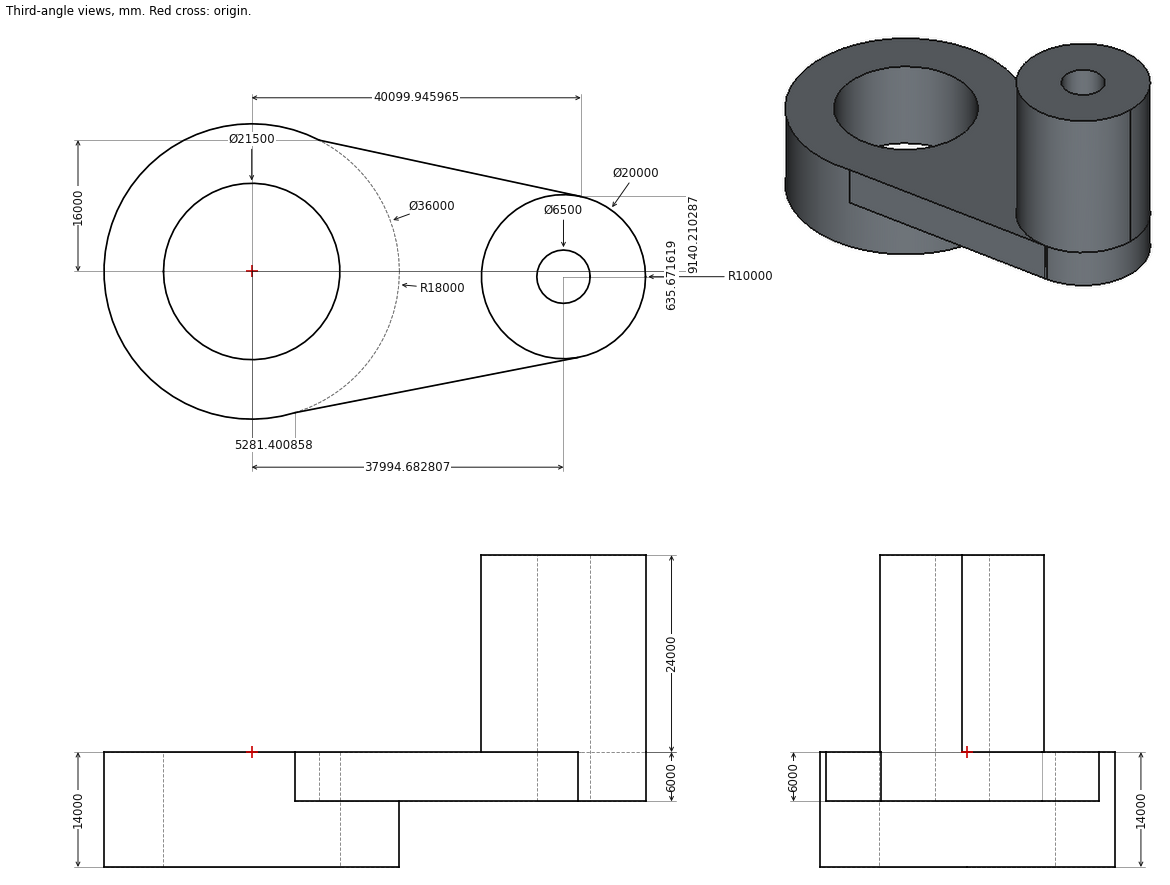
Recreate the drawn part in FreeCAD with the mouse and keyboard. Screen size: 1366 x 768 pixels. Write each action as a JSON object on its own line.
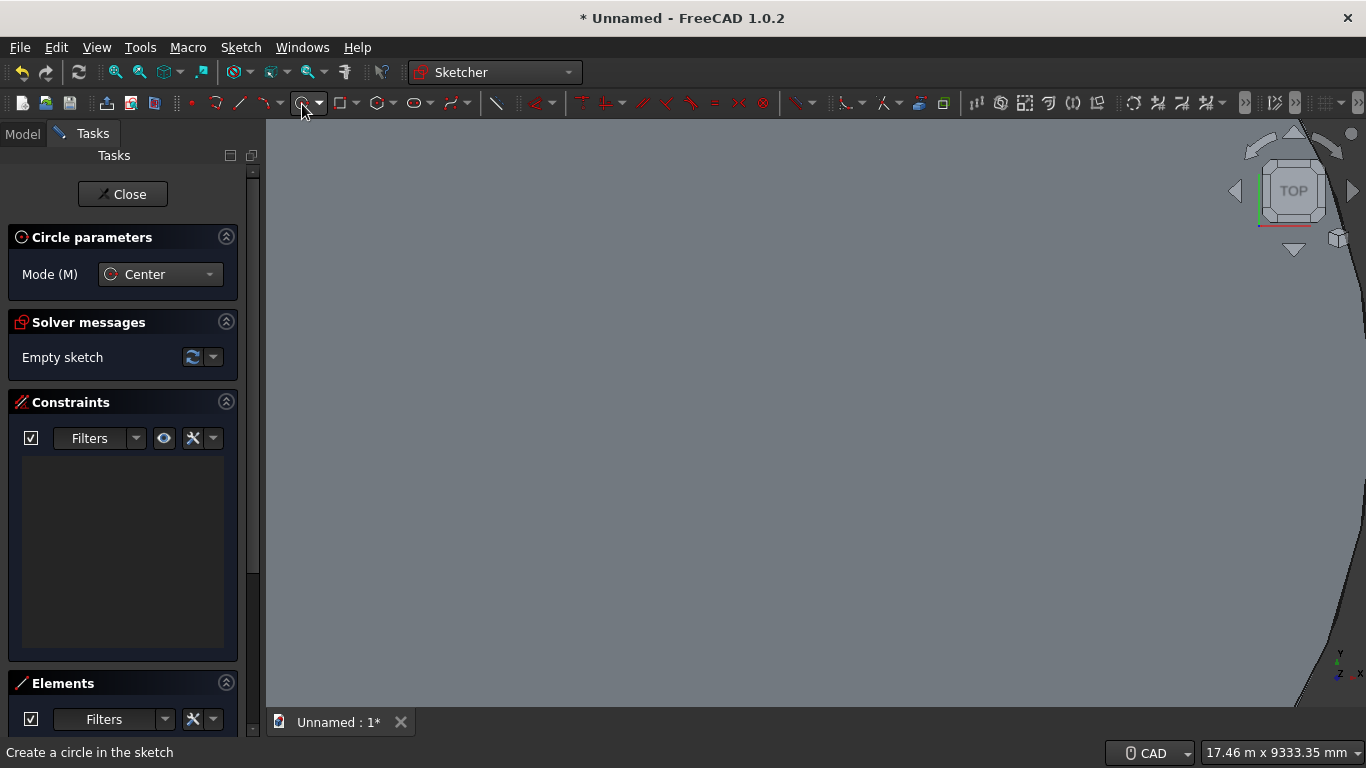
{"action": "left_click", "coordinate": [743, 409]}
{"action": "mouse_move", "coordinate": [887, 264]}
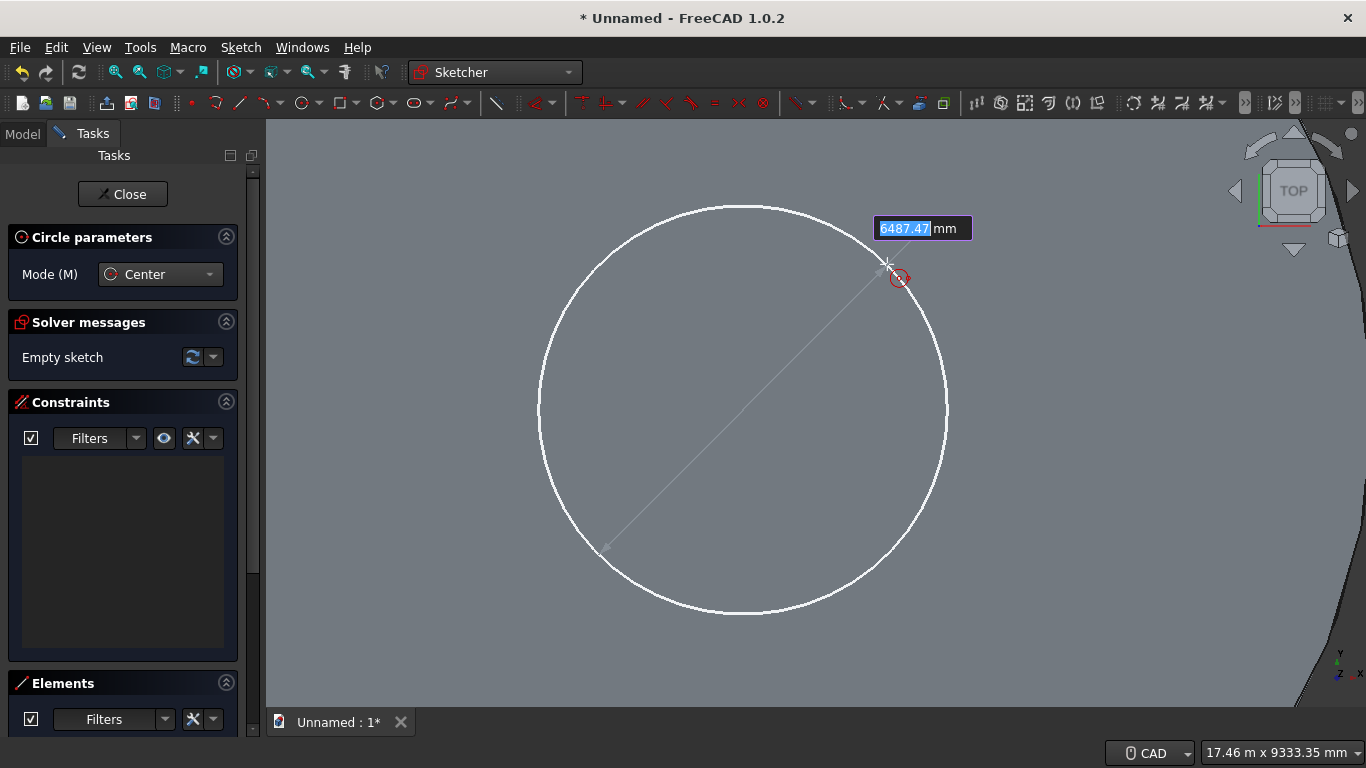
{"action": "type", "text": "6500"}
{"action": "key", "text": "Return"}
{"action": "key", "text": "Escape"}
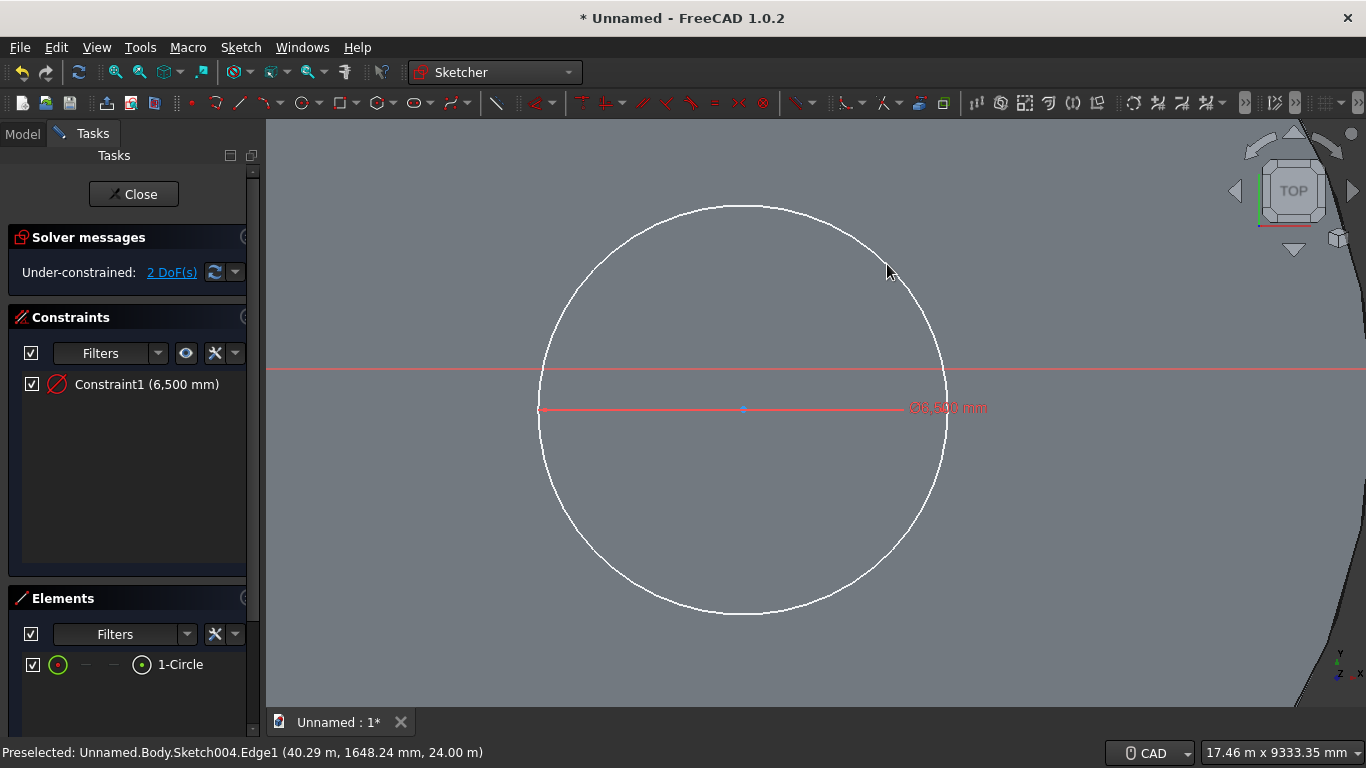
{"action": "left_click", "coordinate": [536, 104]}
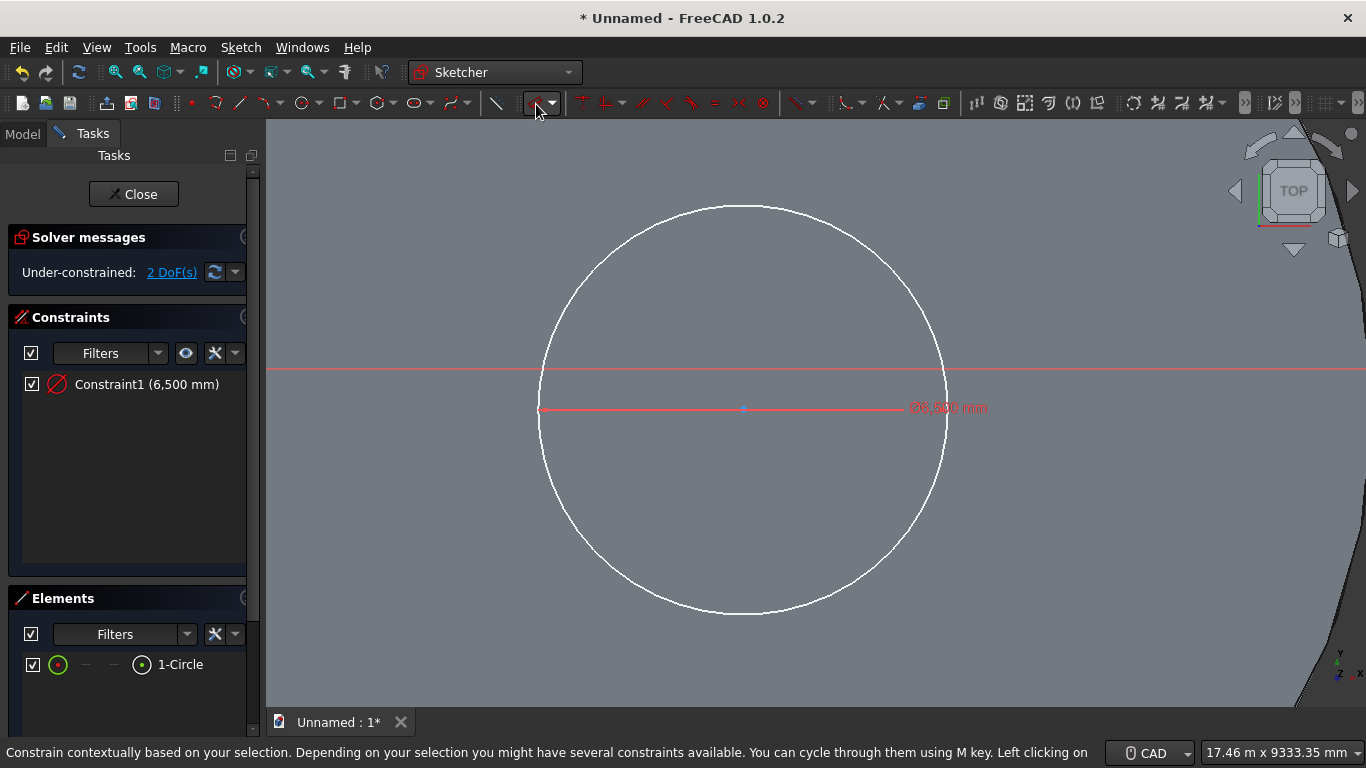
{"action": "left_click", "coordinate": [743, 410]}
{"action": "left_click", "coordinate": [777, 389]}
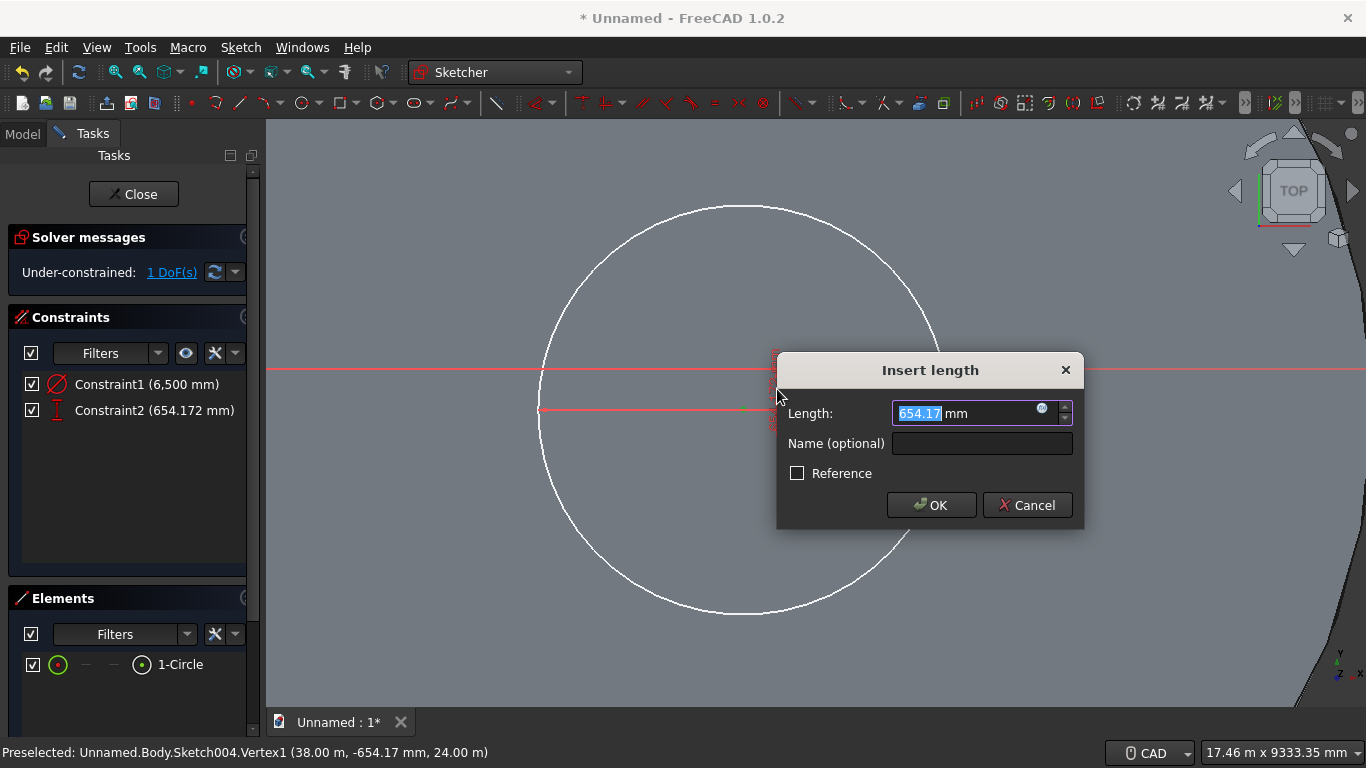
{"action": "type", "text": "635.671619"}
{"action": "key", "text": "Return"}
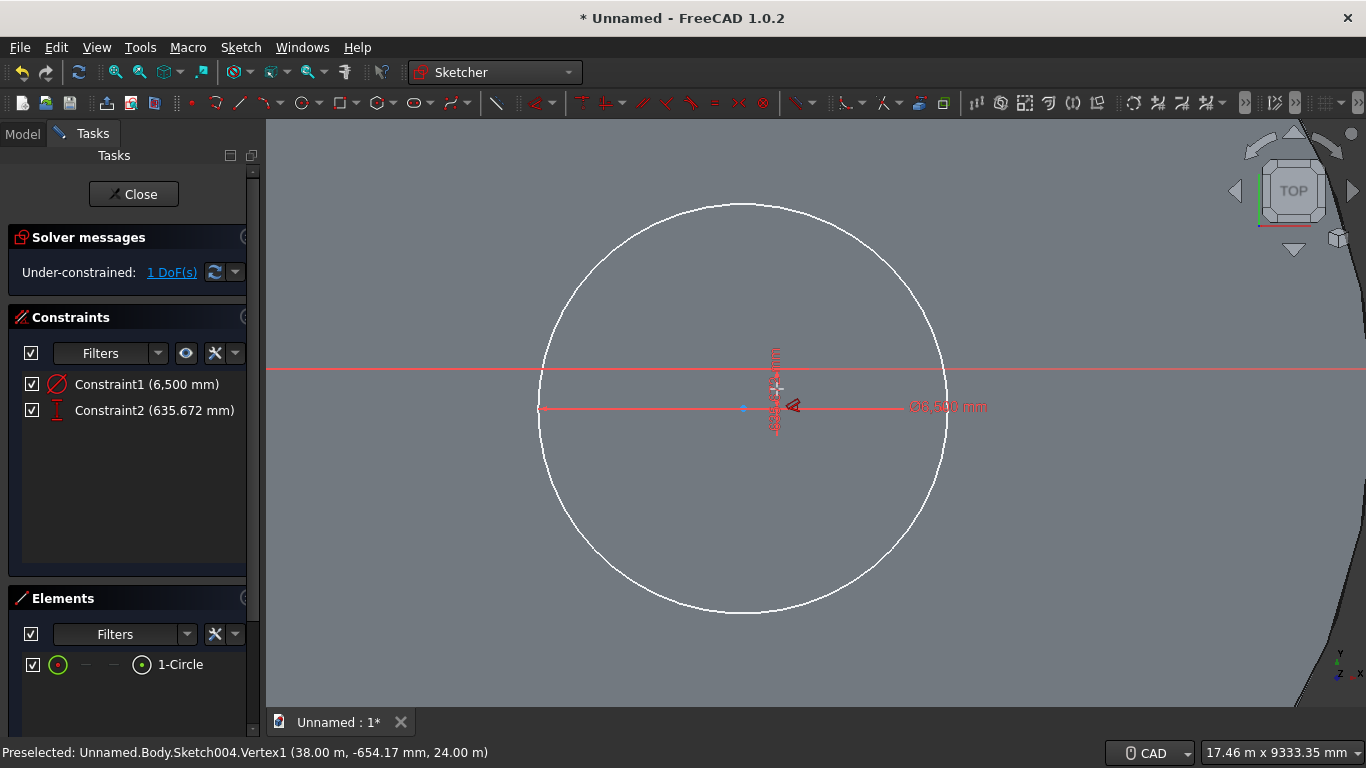
{"action": "left_click", "coordinate": [743, 409]}
{"action": "left_click", "coordinate": [519, 335]}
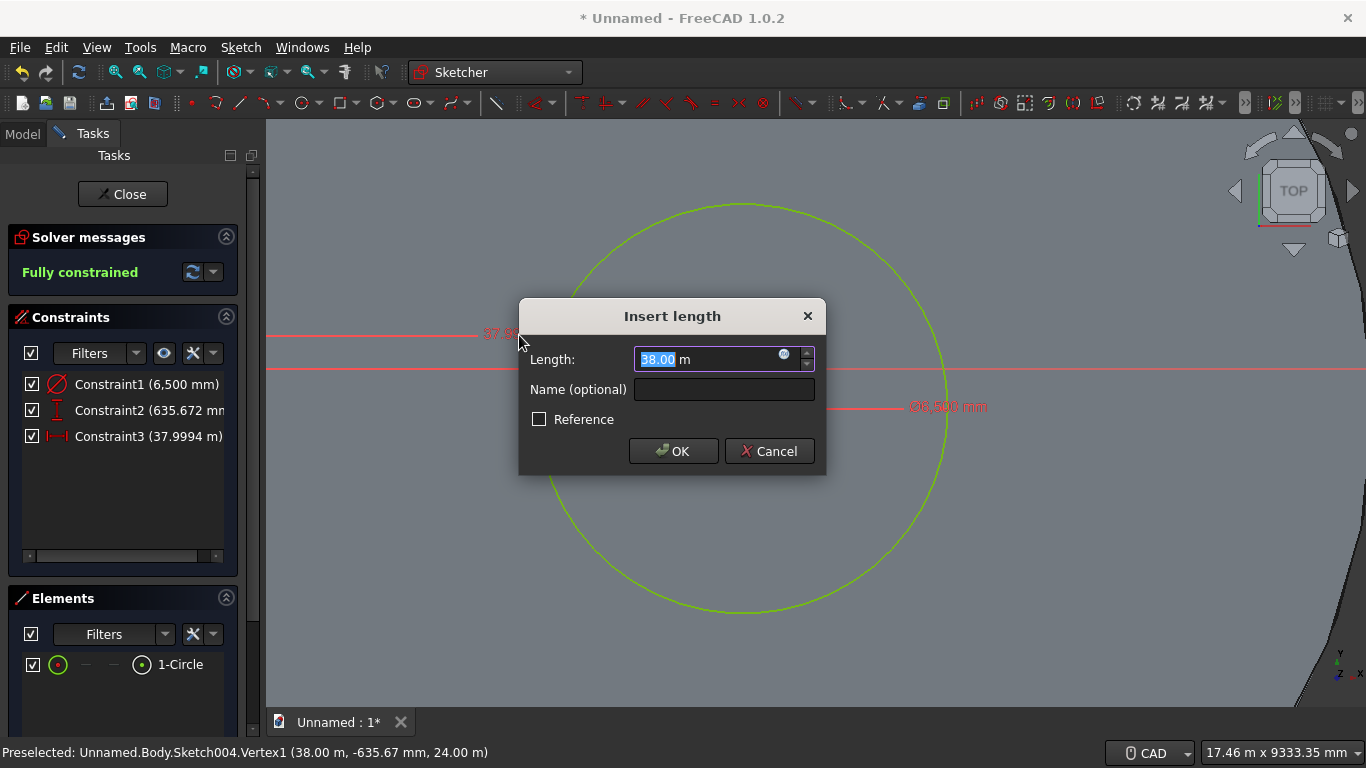
{"action": "key", "text": "ctrl+a"}
{"action": "type", "text": "37994.682807 mm"}
{"action": "key", "text": "Return"}
{"action": "key", "text": "Escape"}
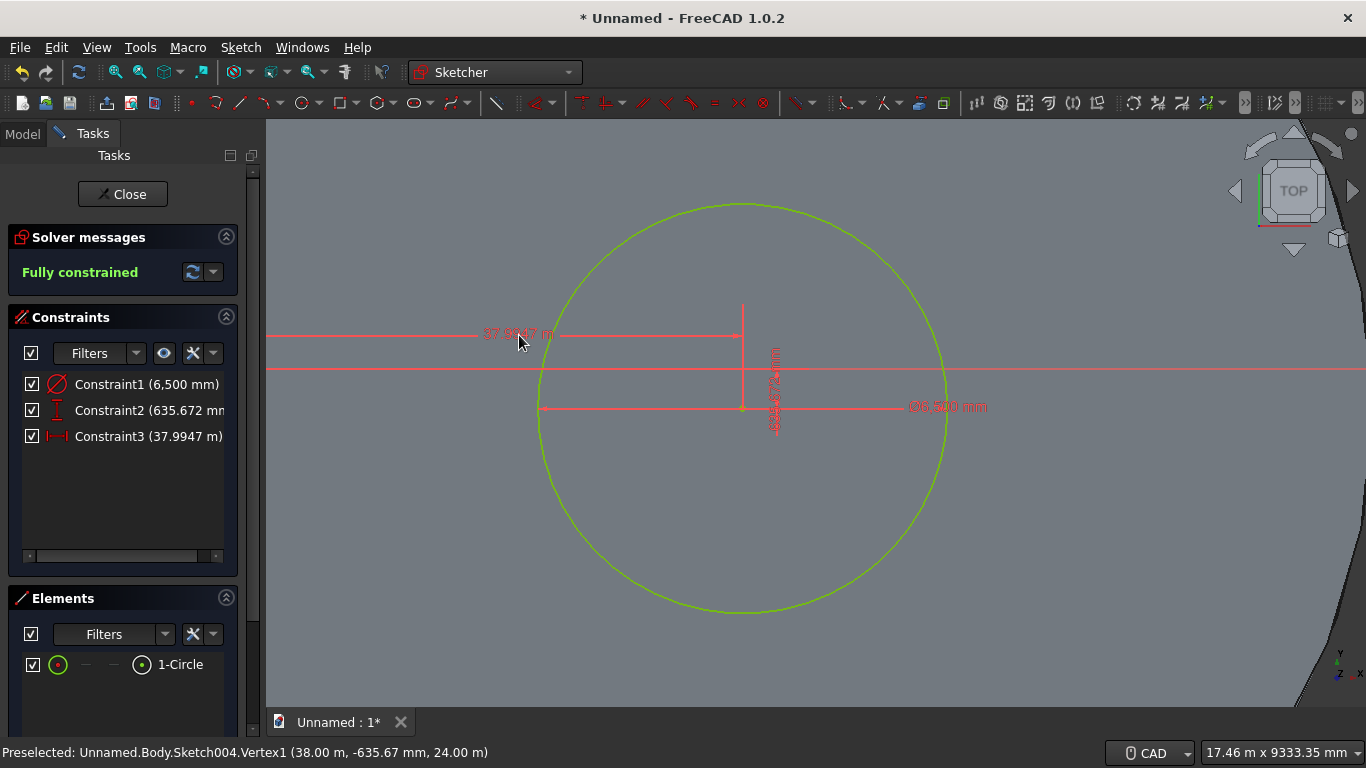
{"action": "left_click", "coordinate": [123, 194]}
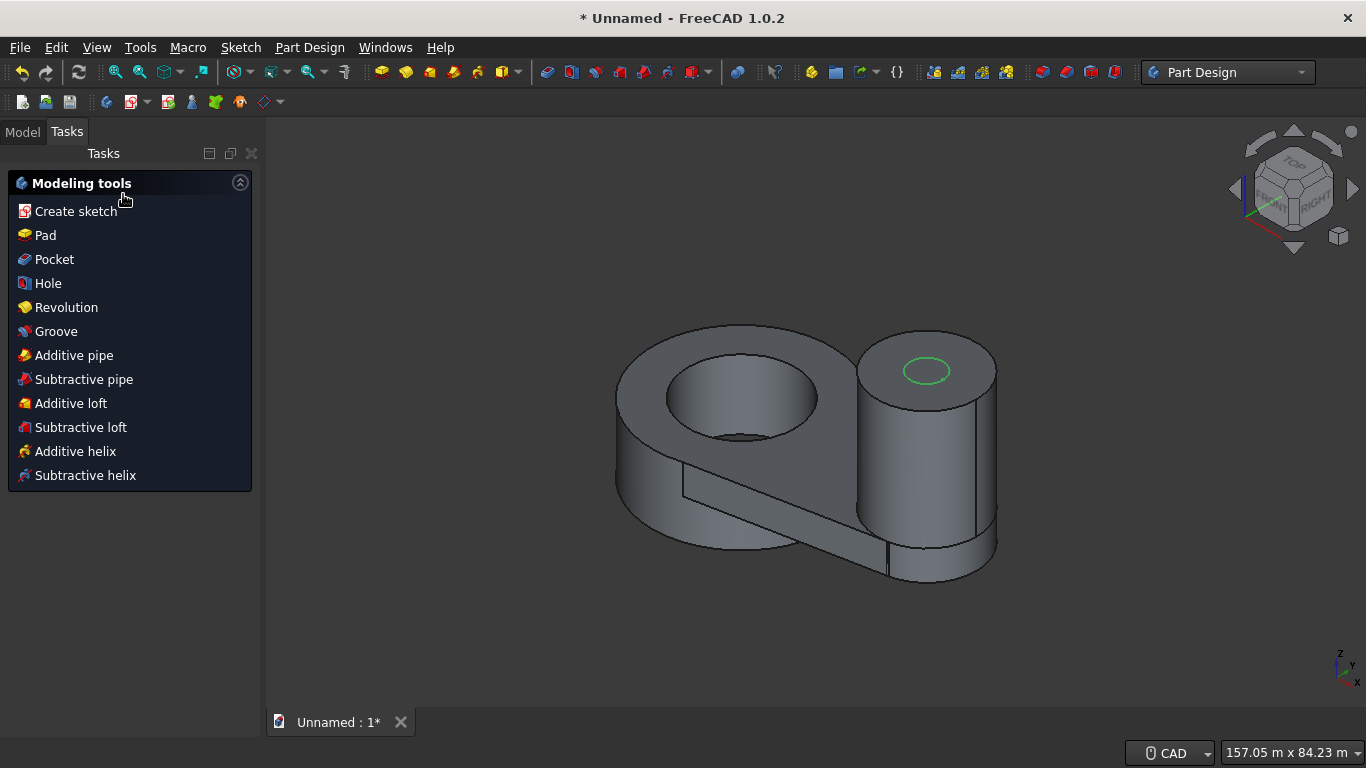
{"action": "left_click", "coordinate": [548, 72]}